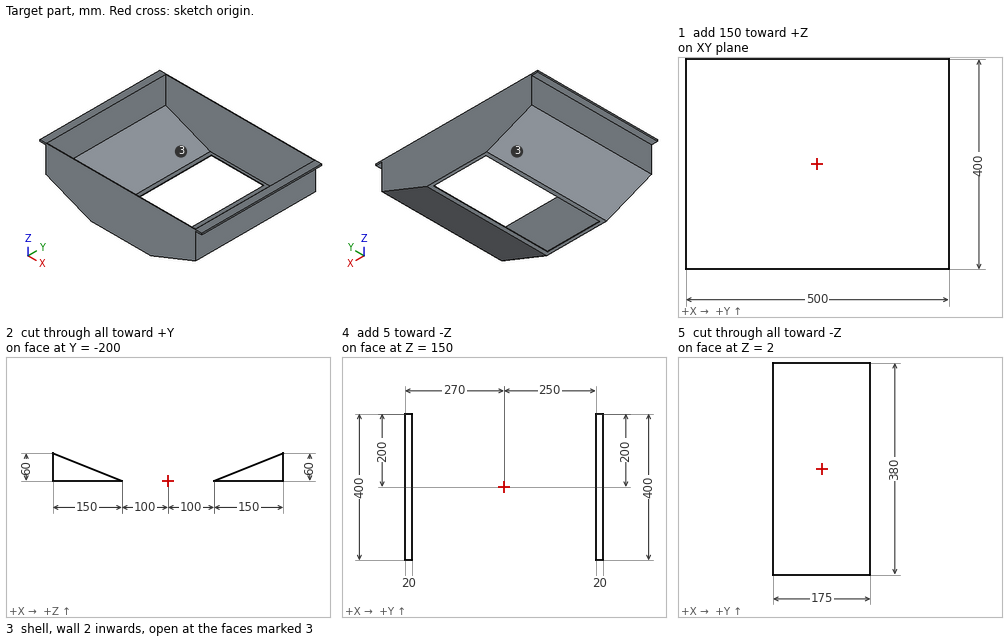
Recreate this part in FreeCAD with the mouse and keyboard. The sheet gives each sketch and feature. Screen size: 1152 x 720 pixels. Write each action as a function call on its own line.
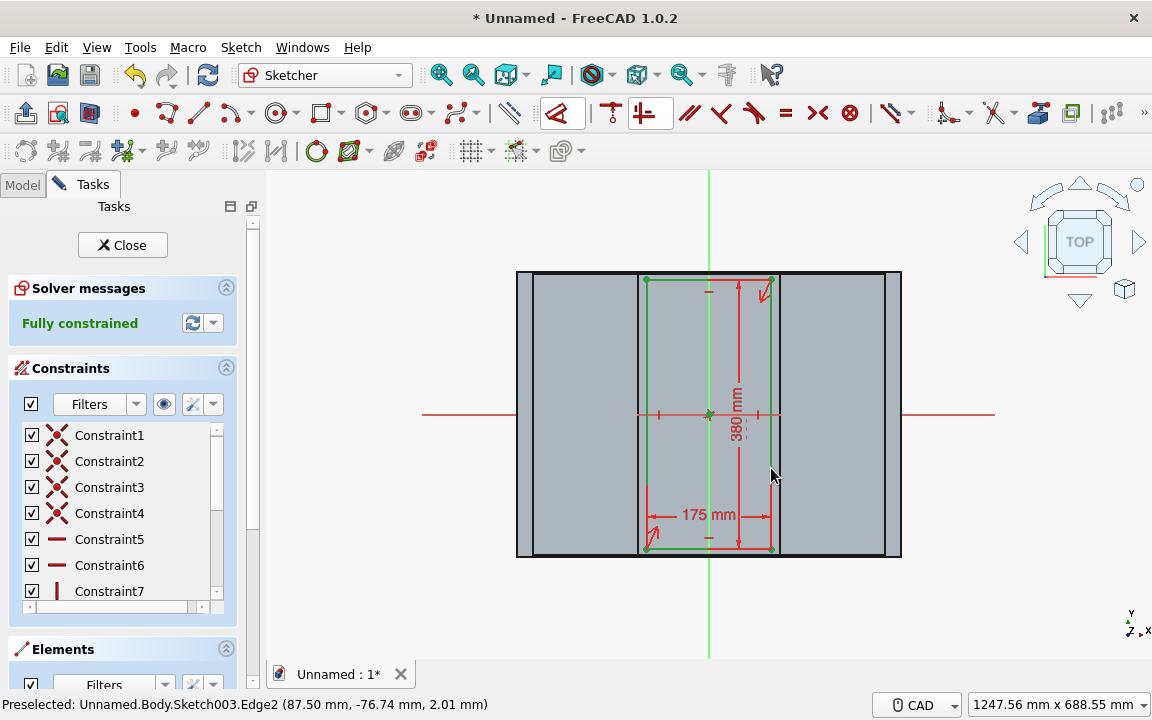
click(123, 245)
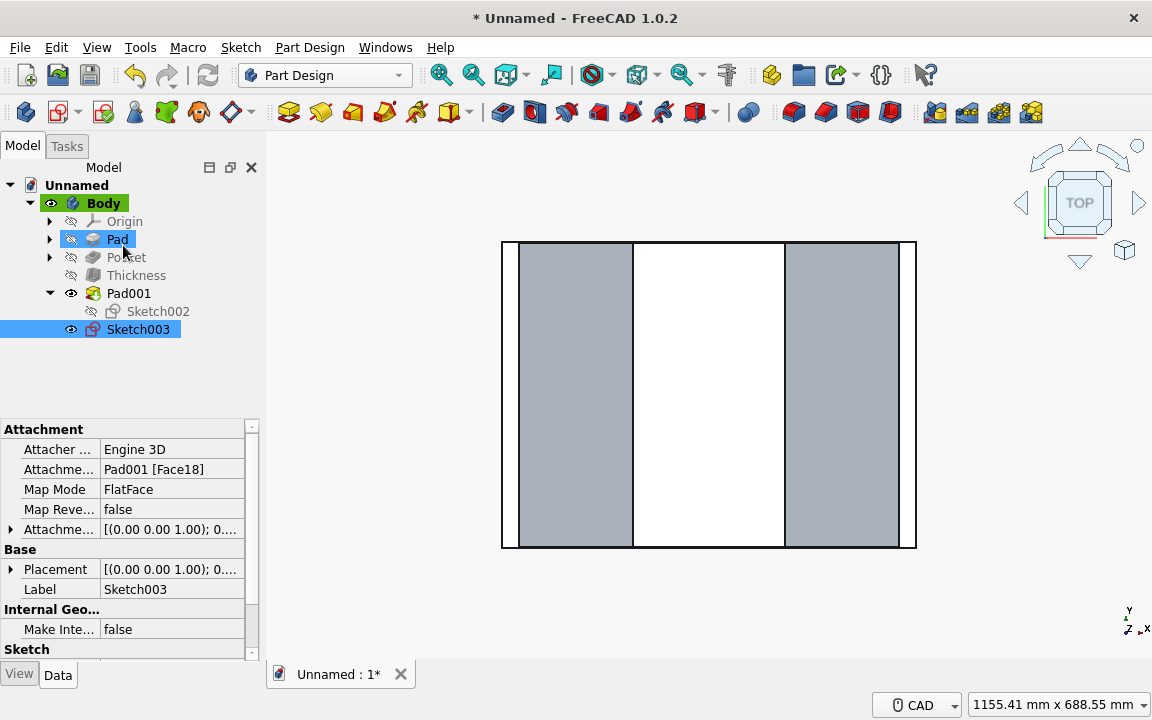
click(504, 112)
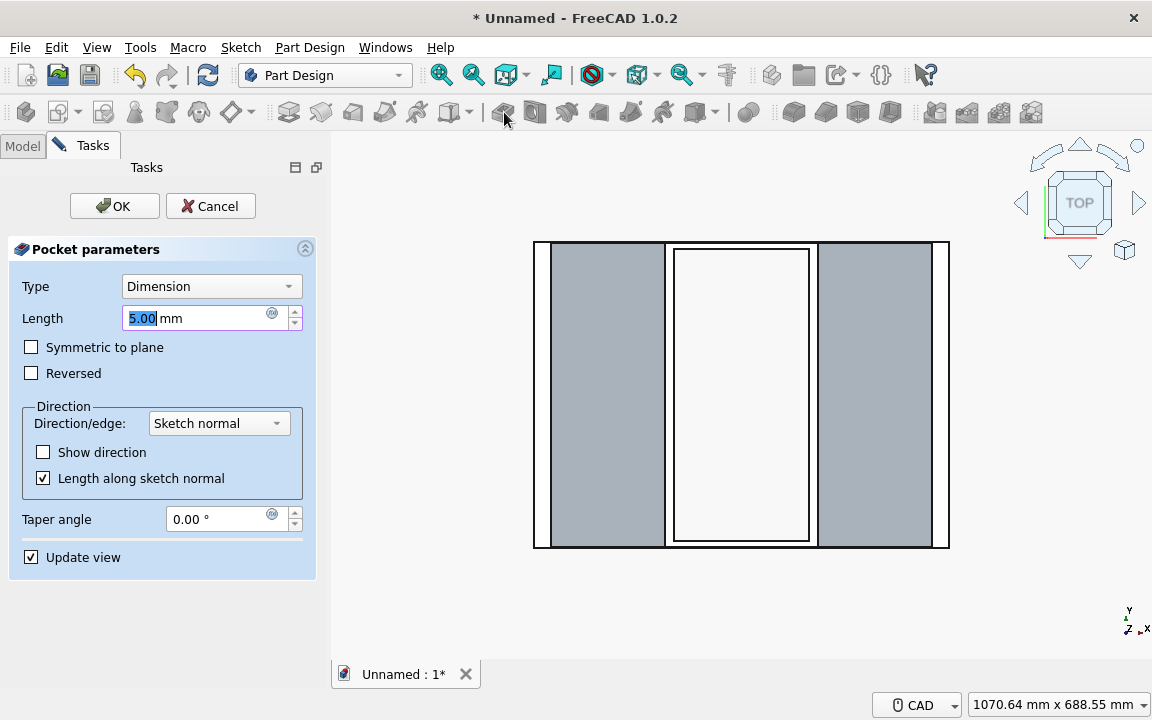
click(212, 286)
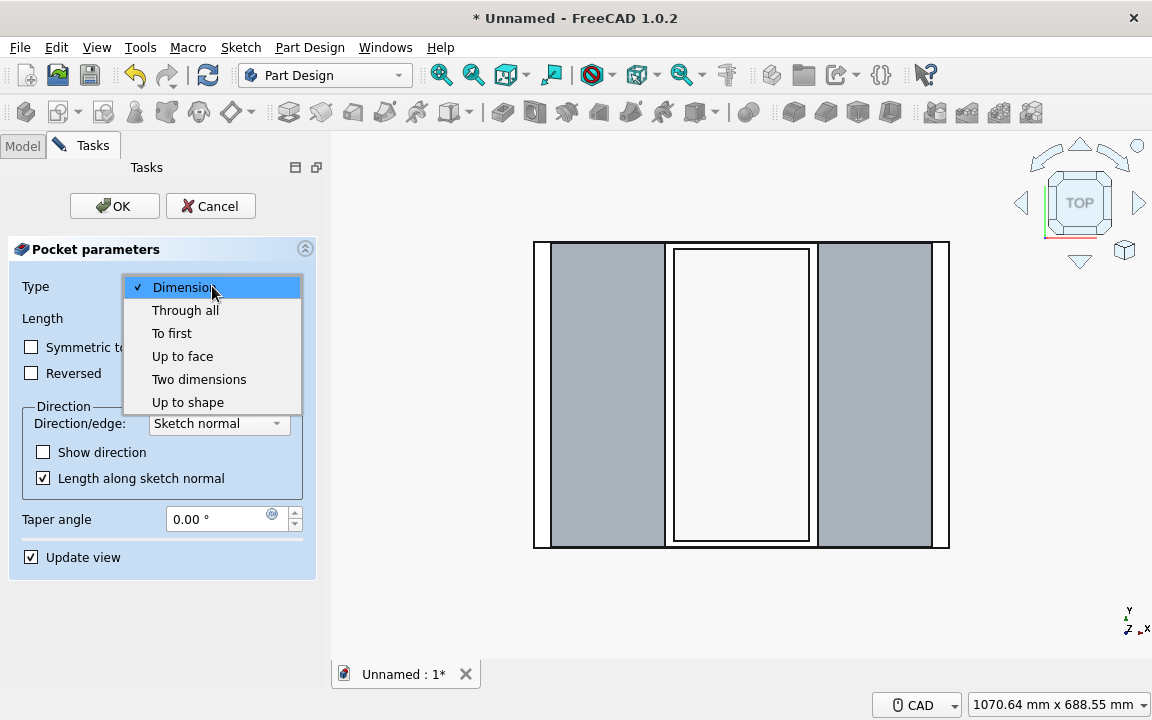
click(212, 310)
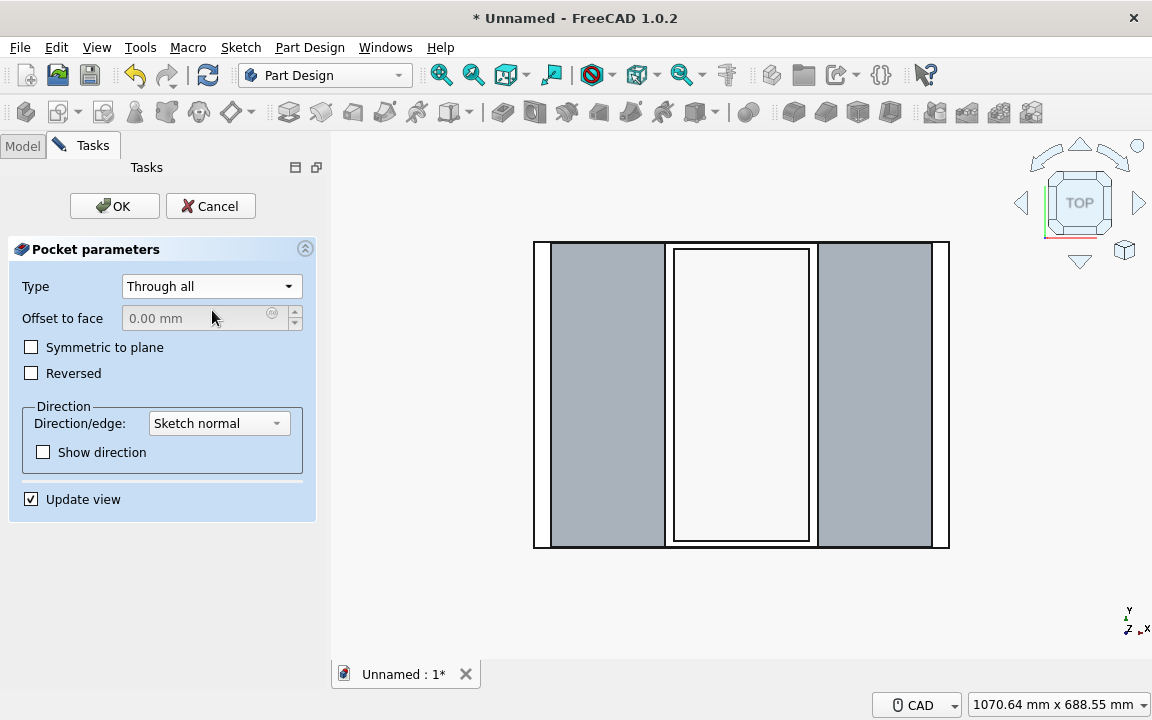
click(115, 206)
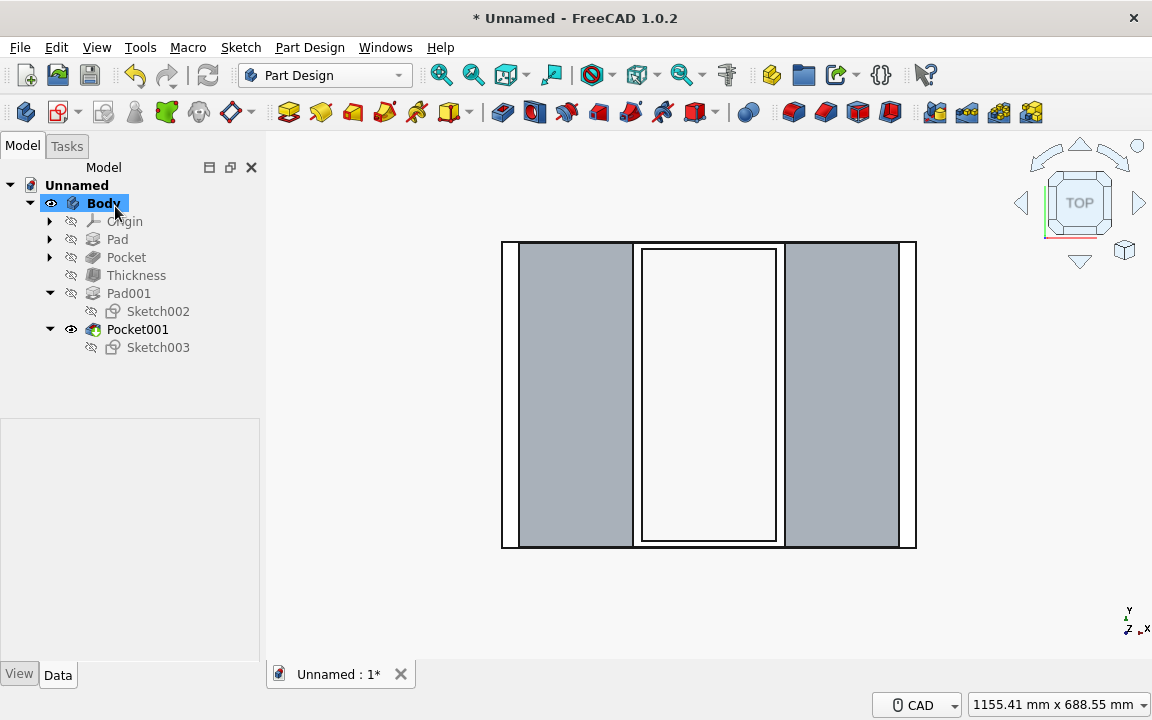
key(0)